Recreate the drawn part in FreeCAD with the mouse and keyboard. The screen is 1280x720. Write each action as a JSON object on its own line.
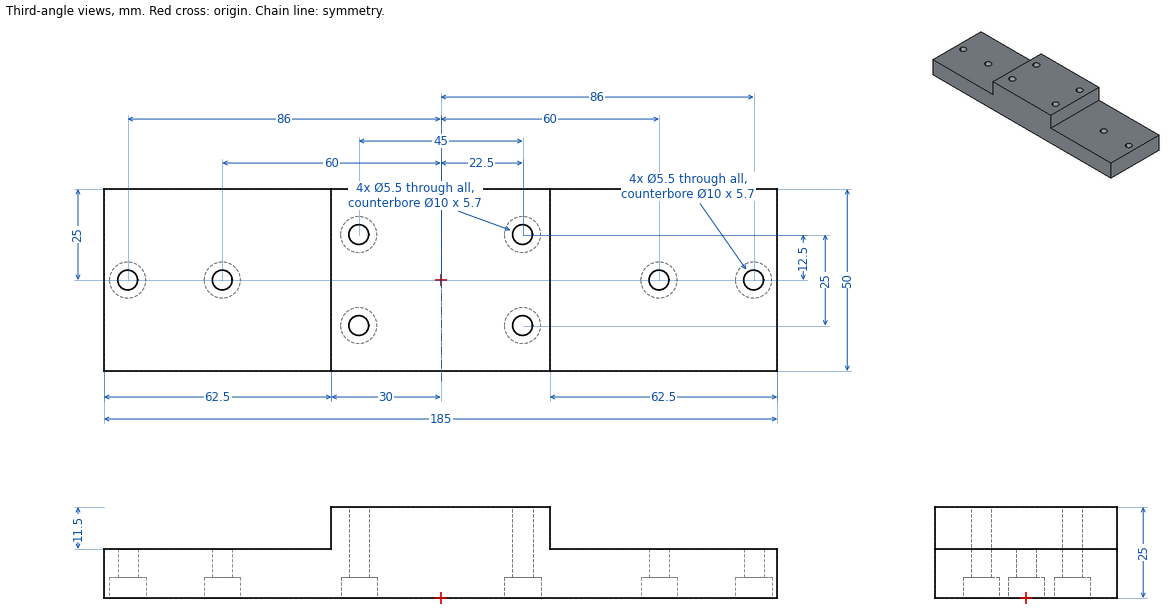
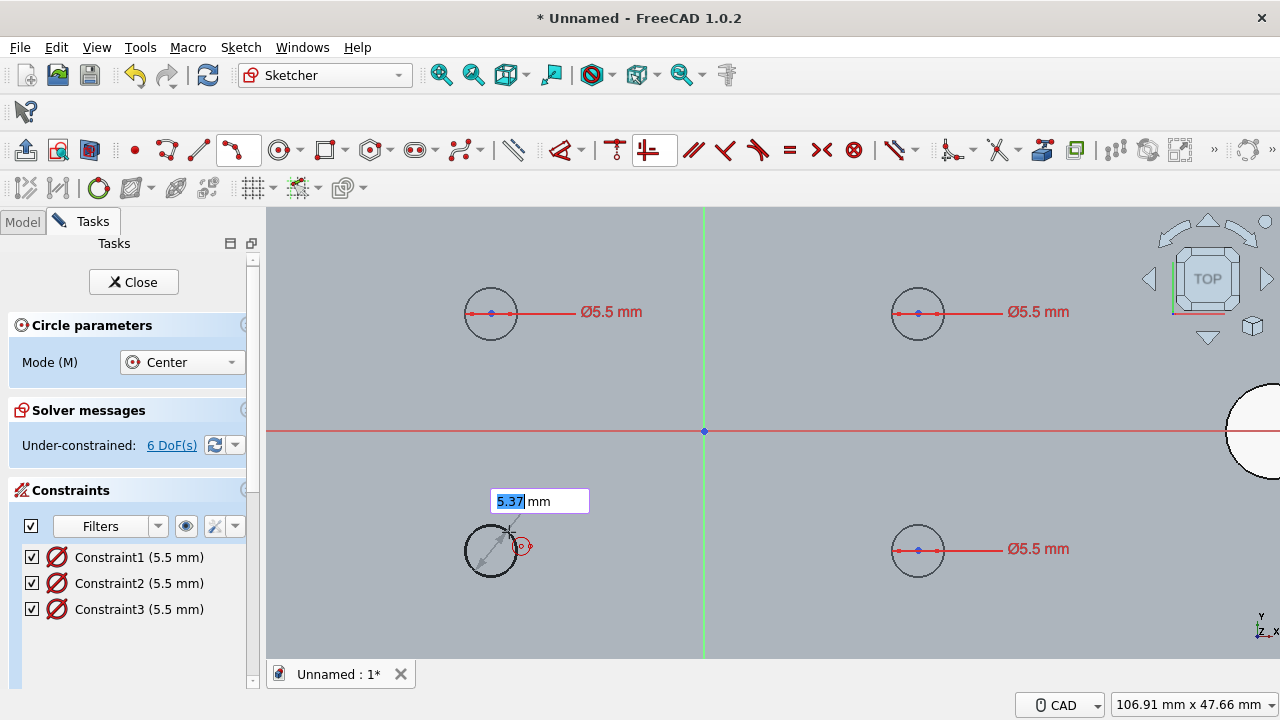
{"action": "type", "text": "5.5"}
{"action": "key", "text": "Return"}
{"action": "key", "text": "Escape"}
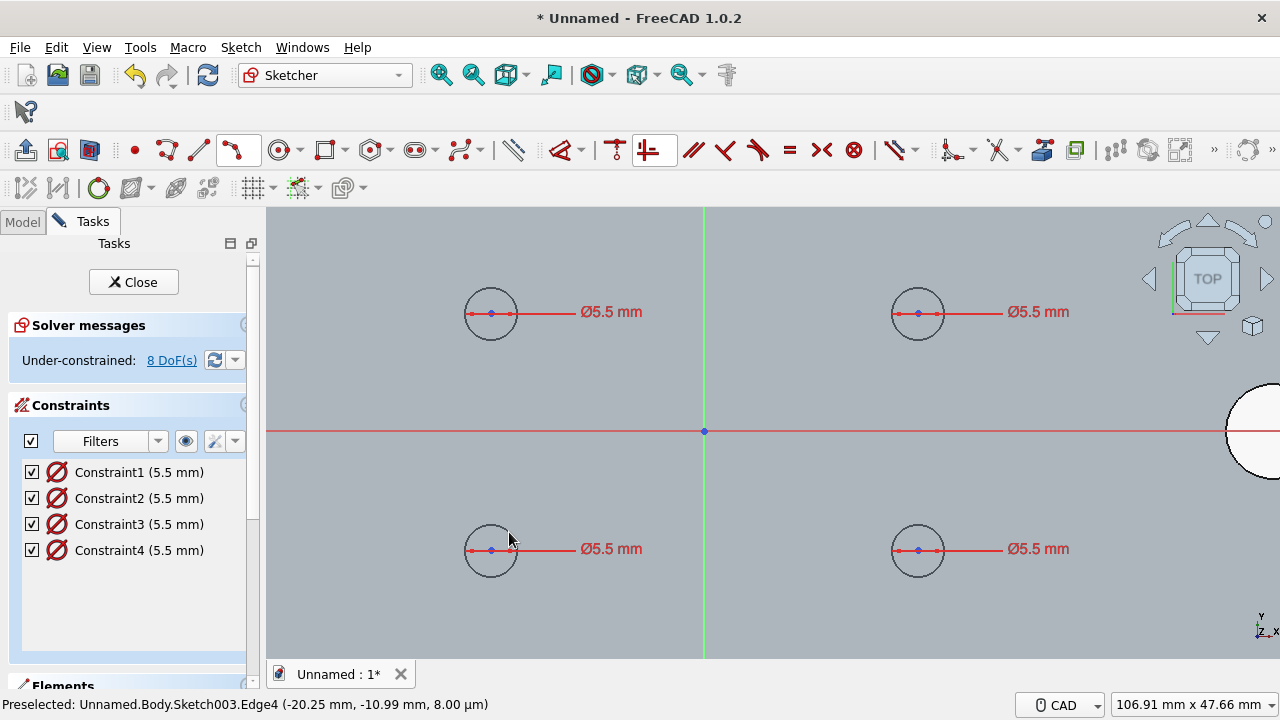
{"action": "left_click", "coordinate": [918, 314]}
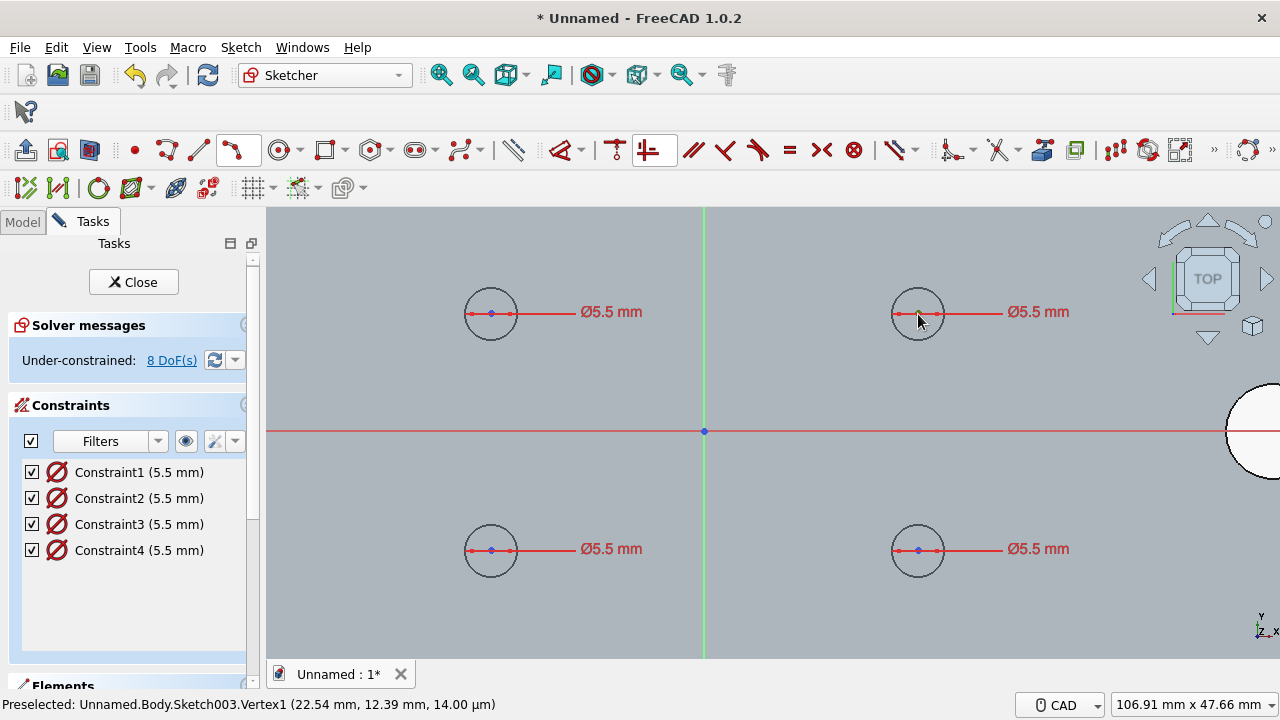
{"action": "left_click", "coordinate": [918, 551]}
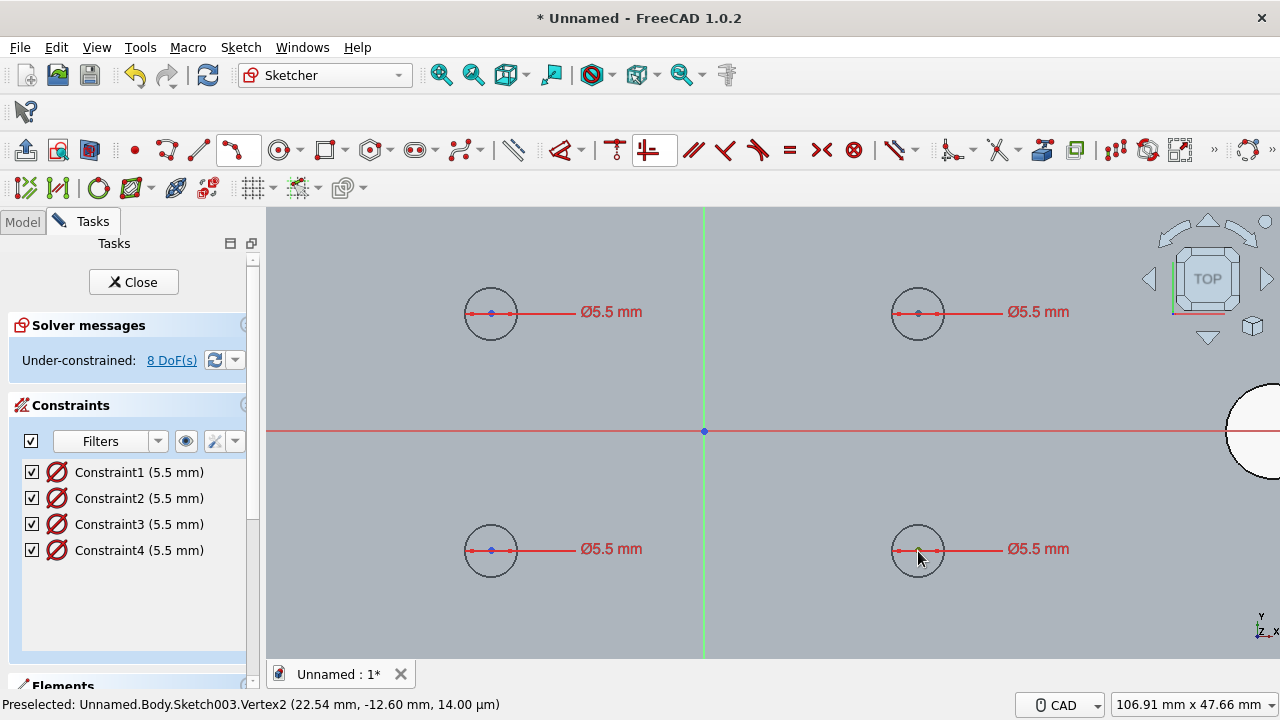
{"action": "key", "text": "v"}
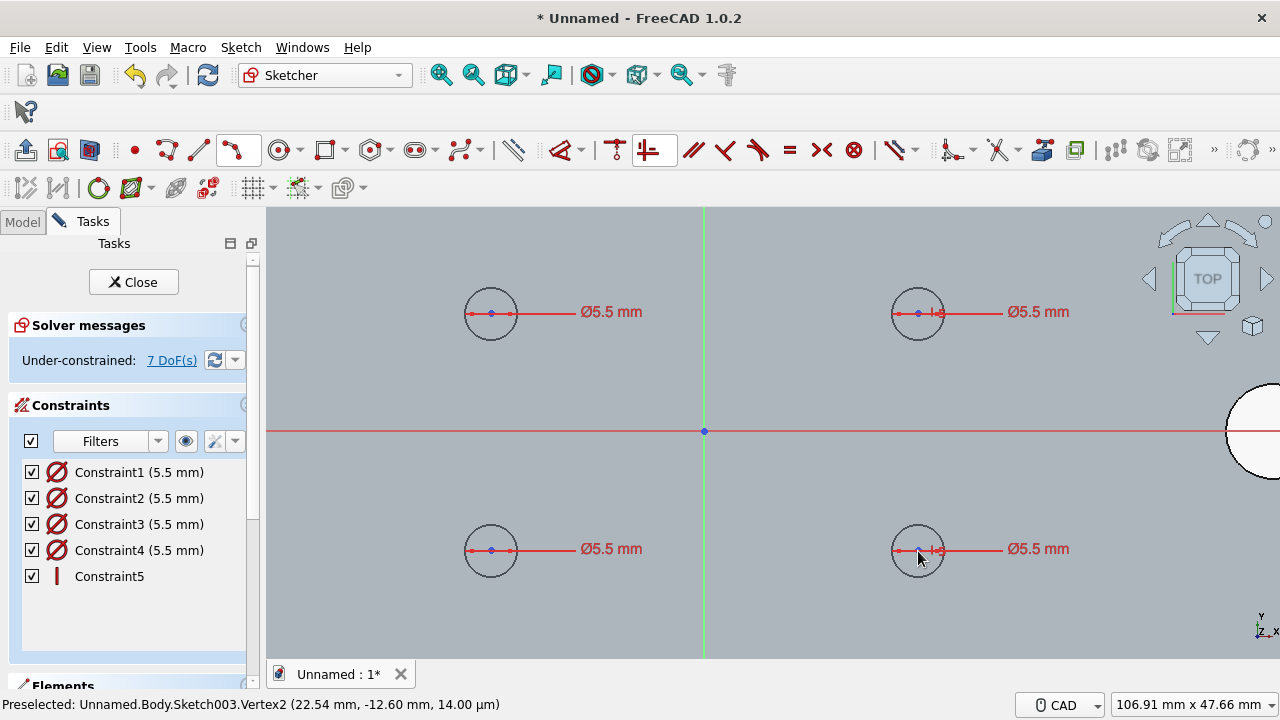
{"action": "left_click", "coordinate": [918, 314]}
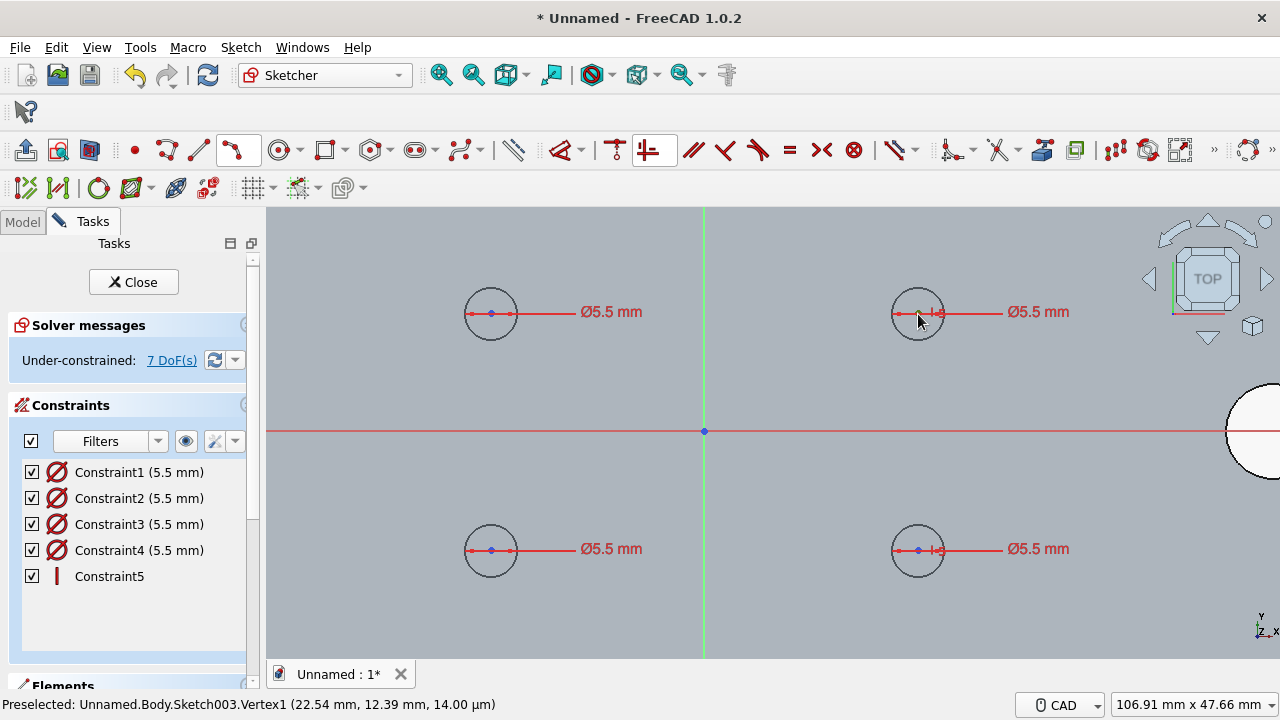
{"action": "left_click", "coordinate": [491, 314]}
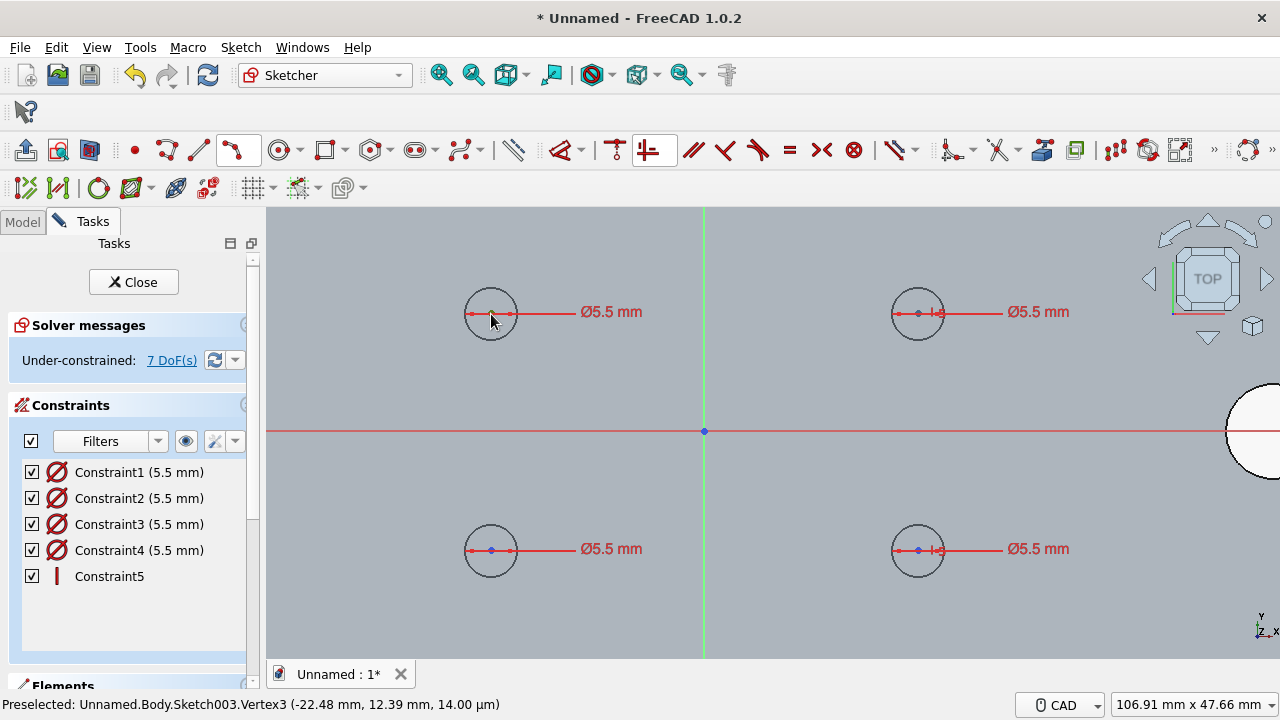
{"action": "left_click", "coordinate": [672, 150]}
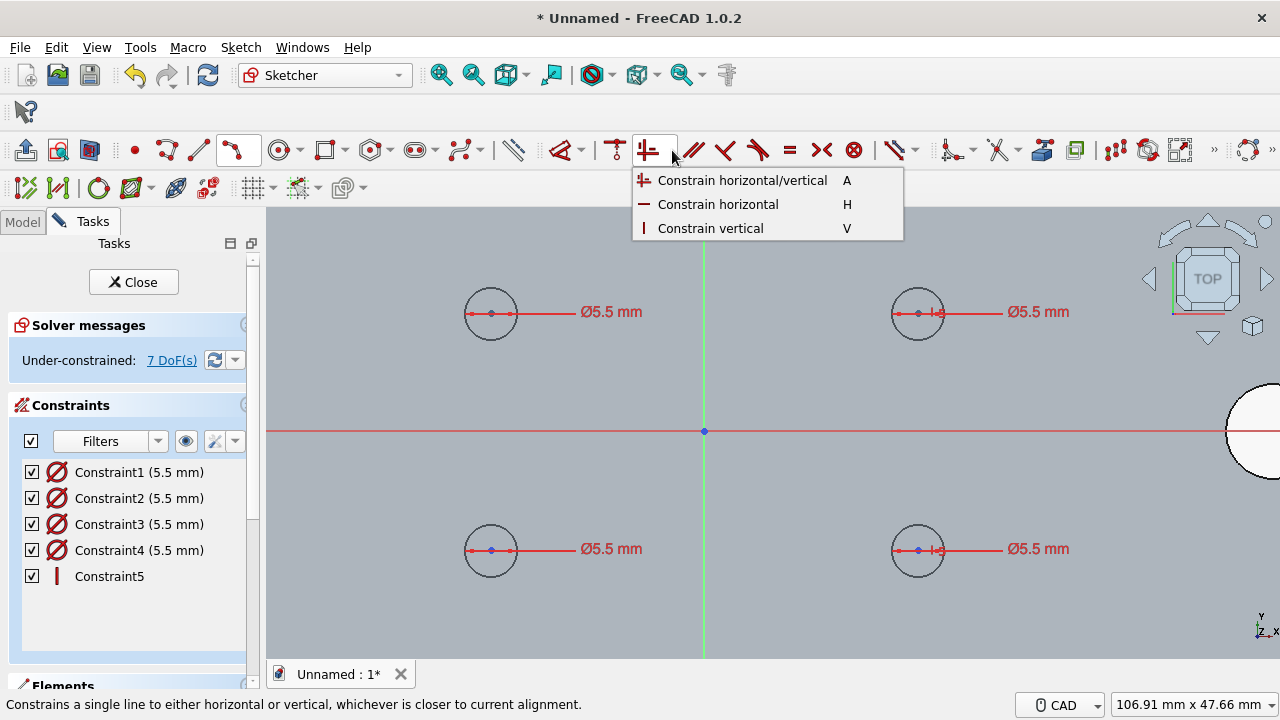
{"action": "left_click", "coordinate": [768, 204]}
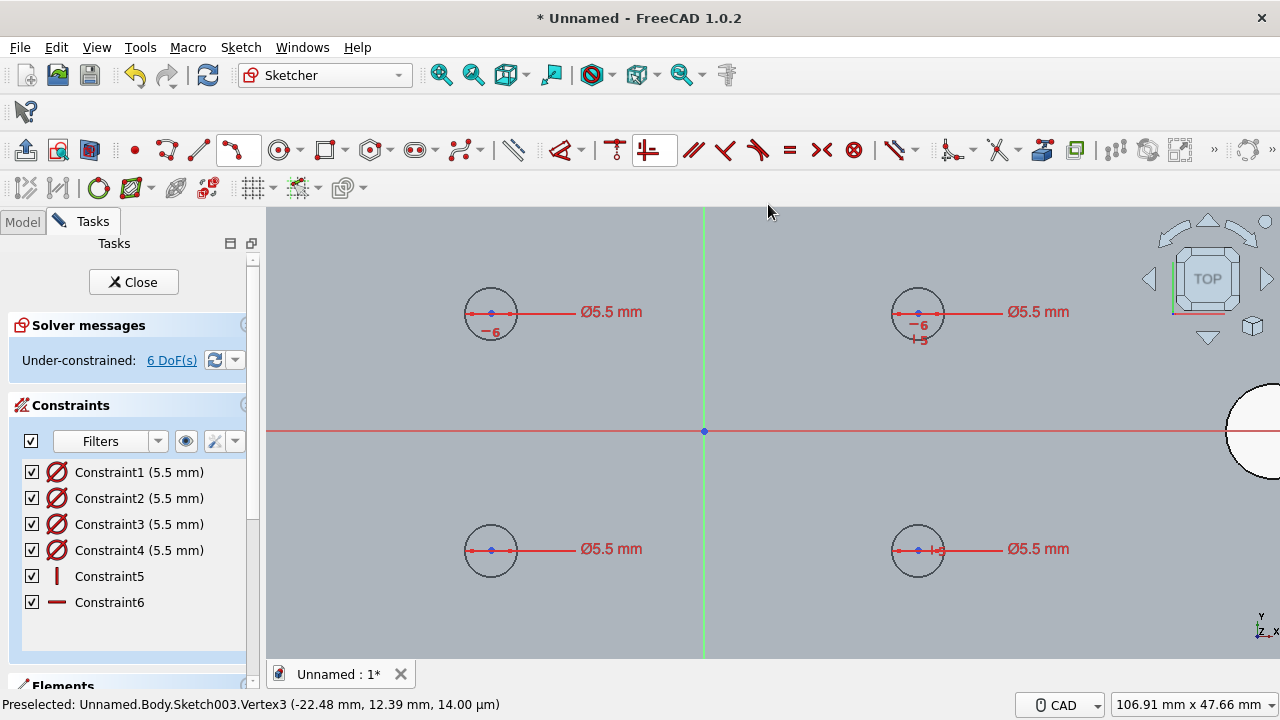
{"action": "left_click", "coordinate": [491, 314]}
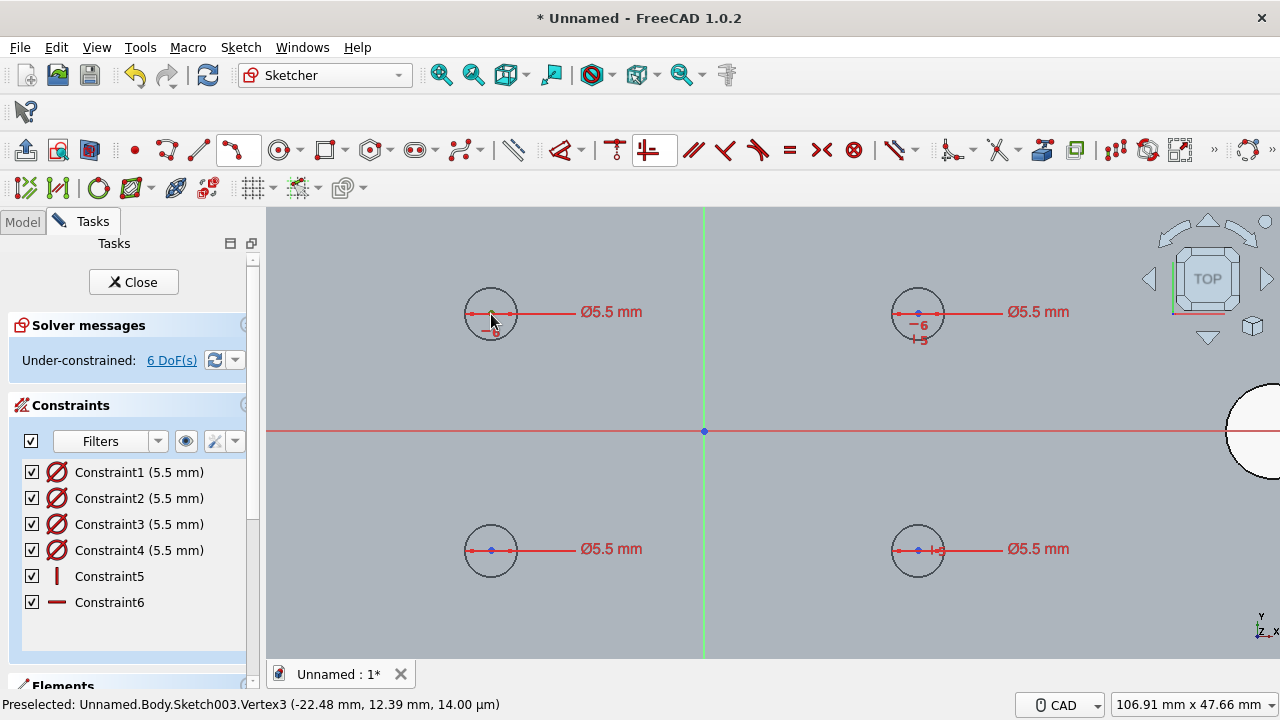
{"action": "left_click", "coordinate": [491, 551]}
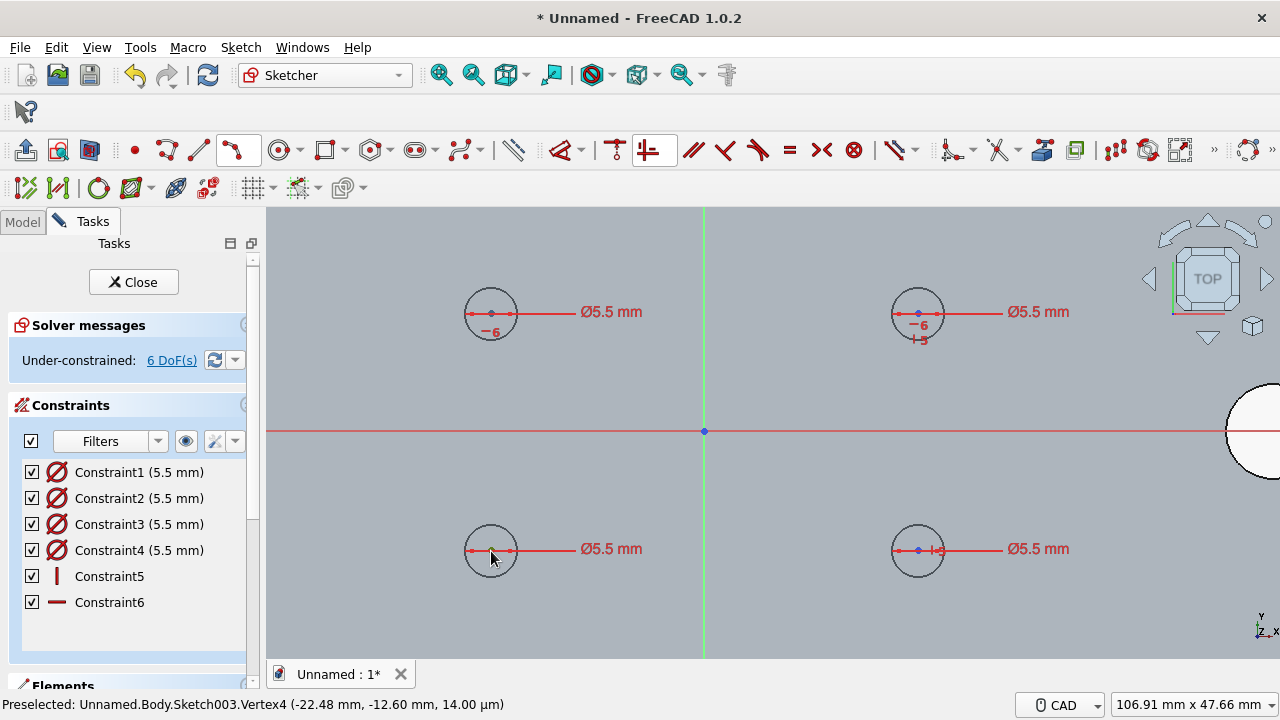
{"action": "left_click", "coordinate": [672, 150]}